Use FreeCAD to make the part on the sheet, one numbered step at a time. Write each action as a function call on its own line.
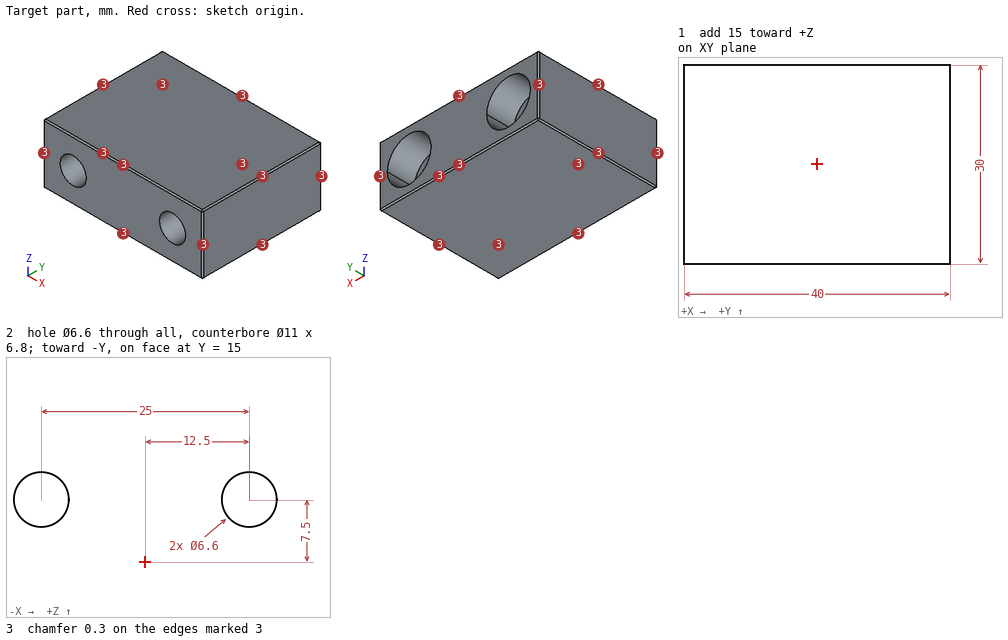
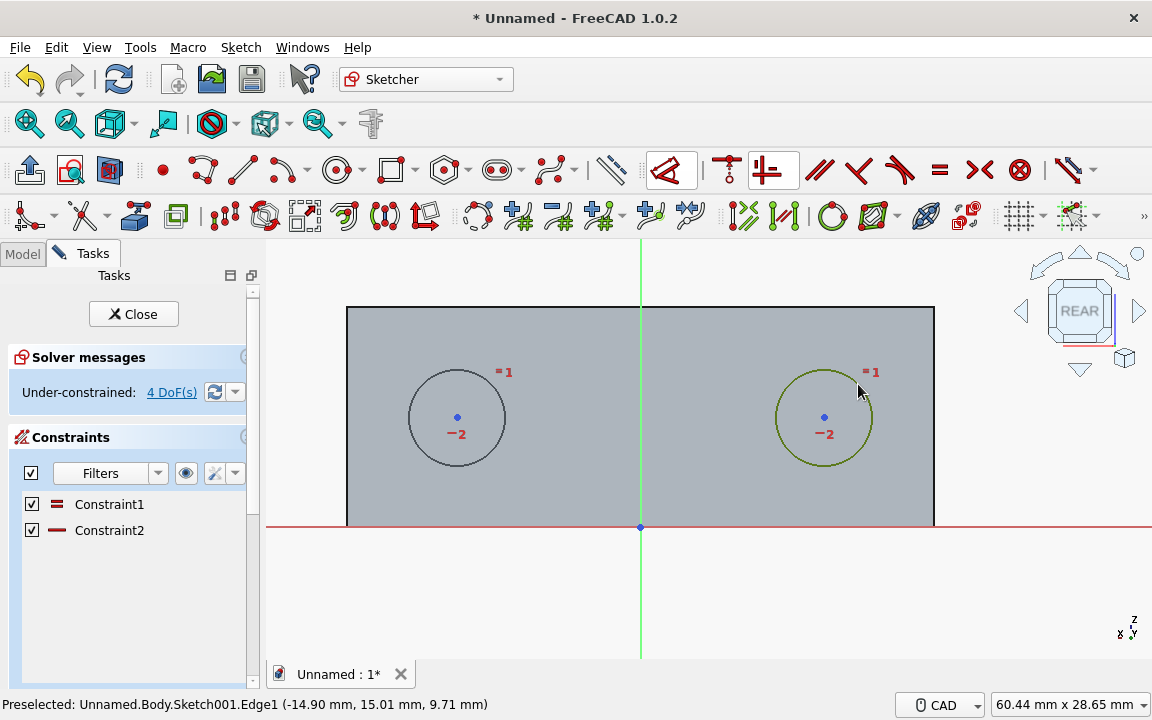
key(k)
key(o)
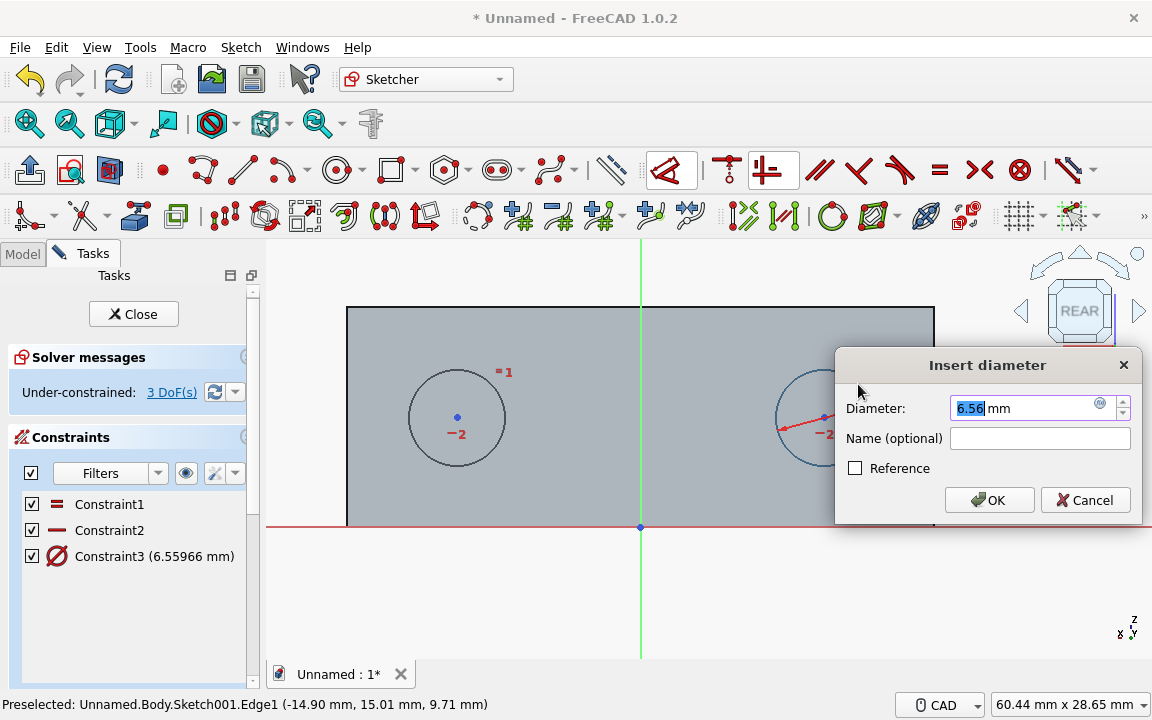
text(6.6)
key(Return)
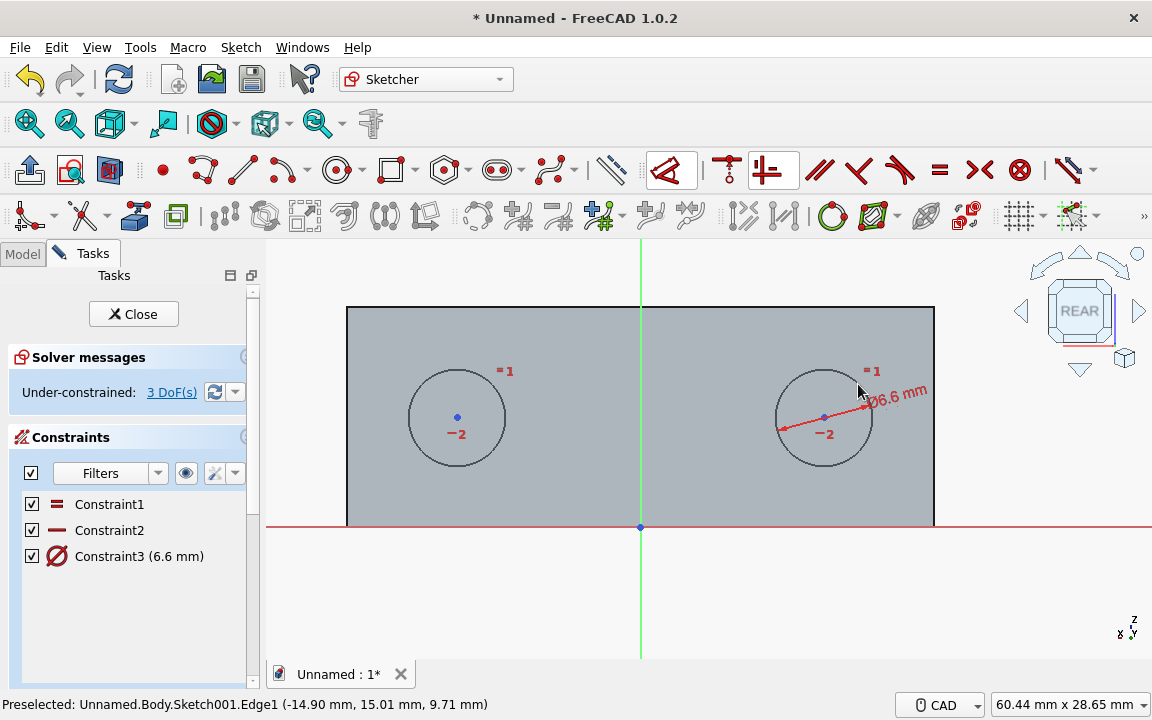
click(824, 418)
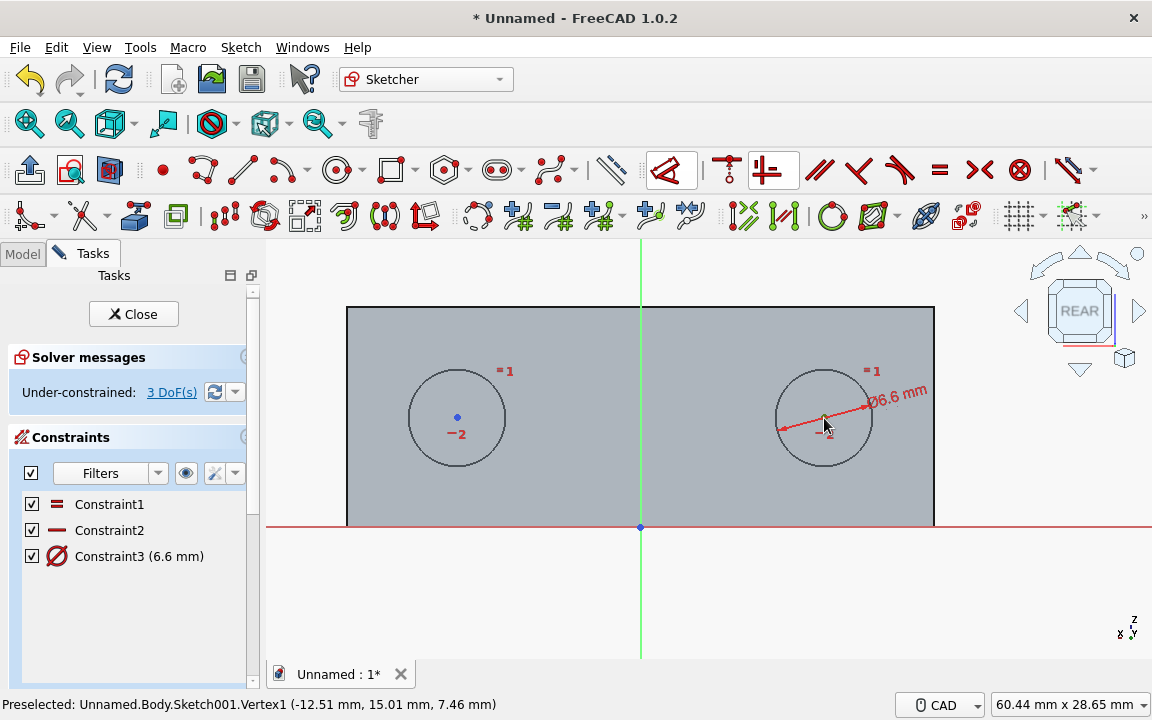
click(692, 170)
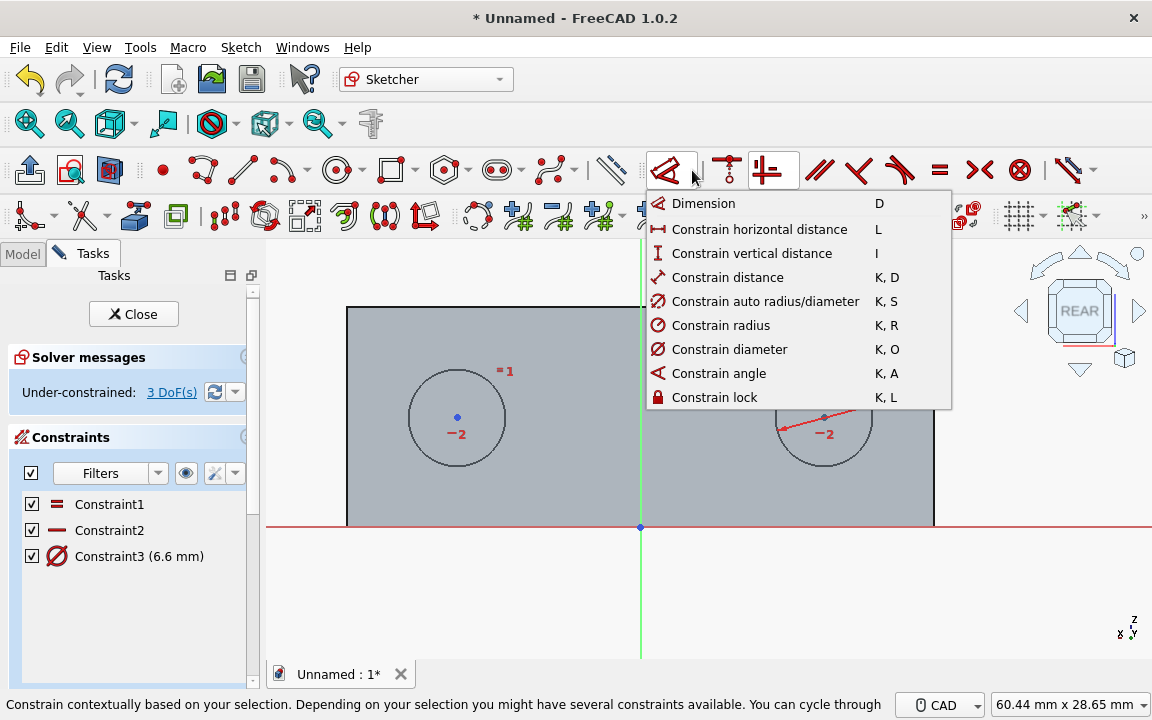
click(799, 253)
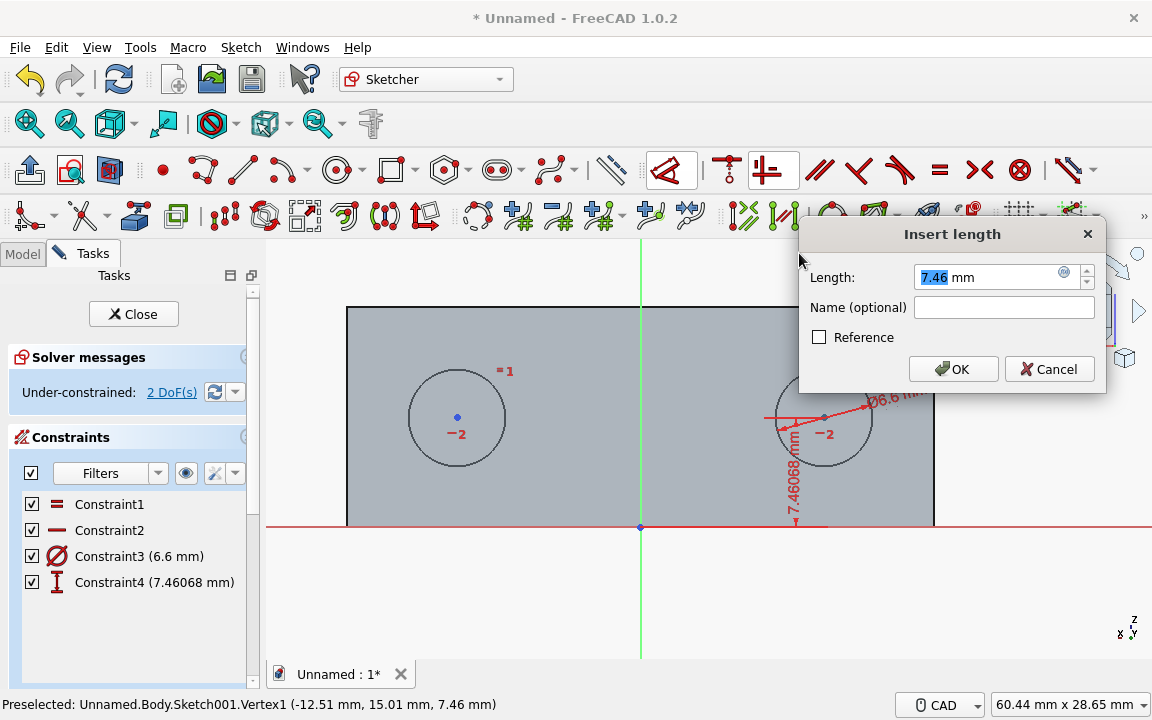
text(7.5)
key(Return)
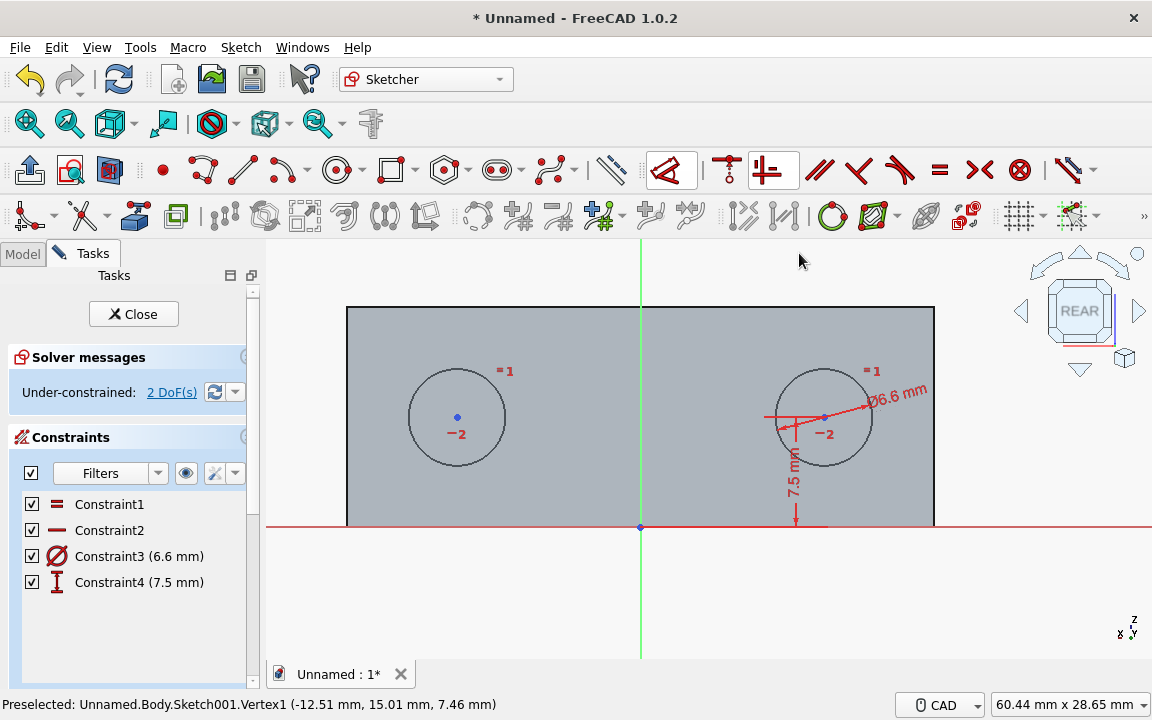
click(824, 417)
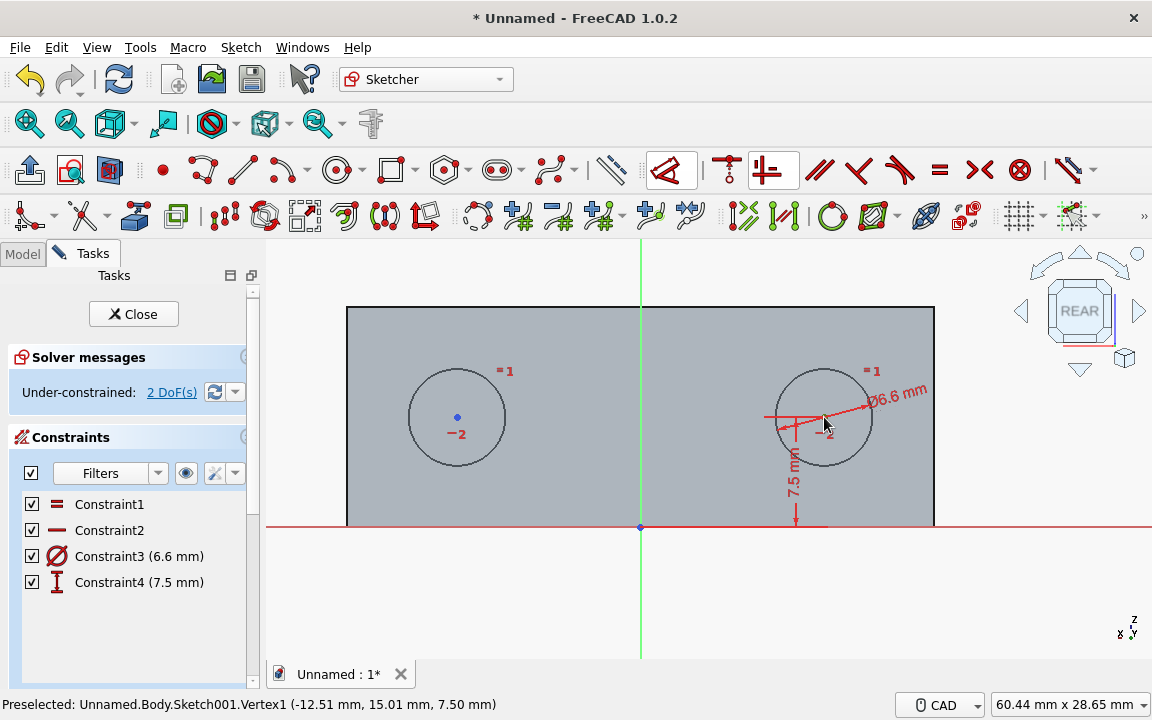
click(457, 417)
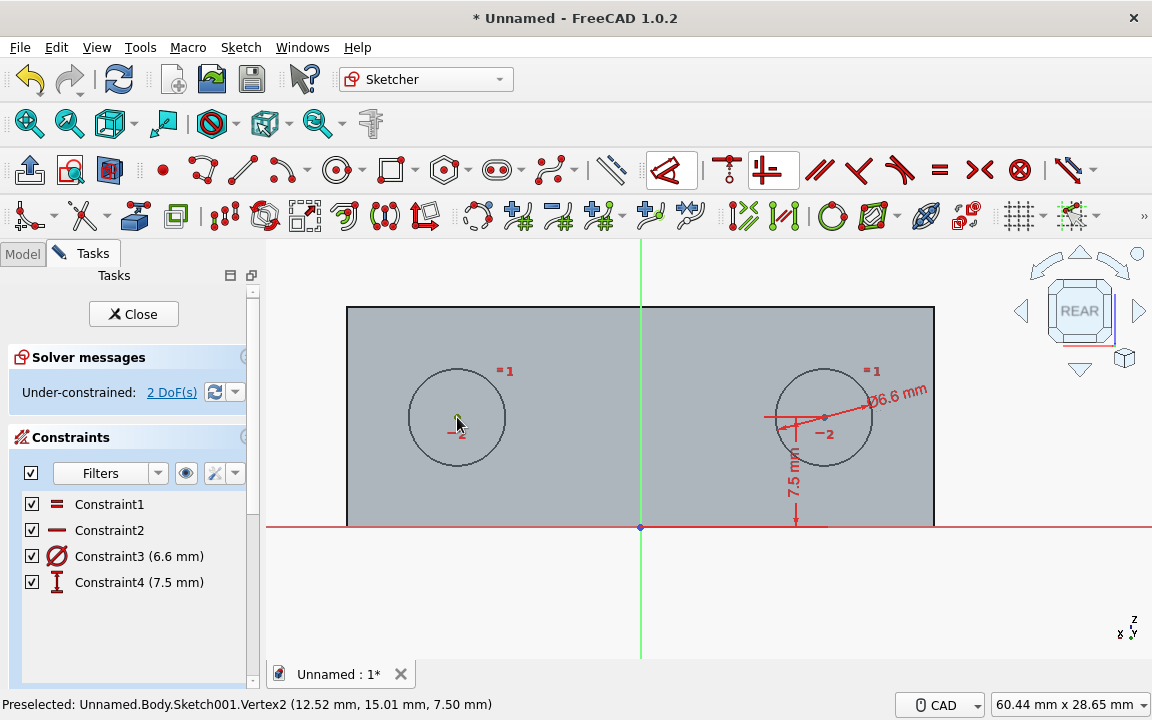
click(692, 170)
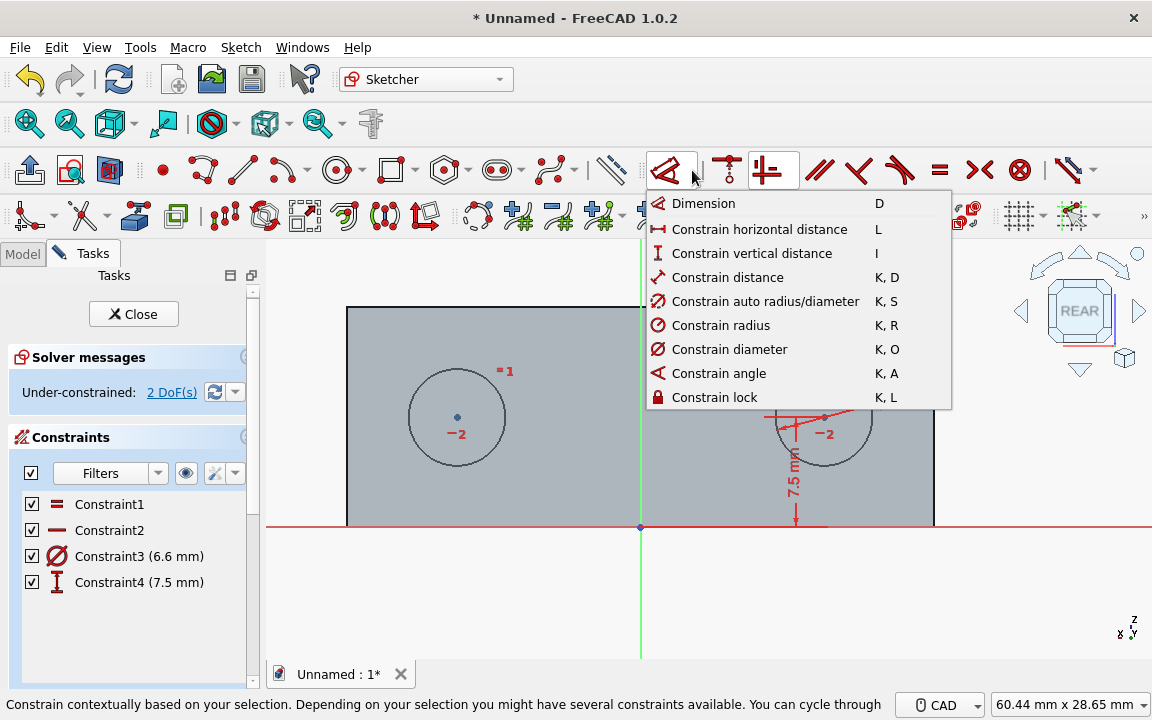
click(799, 229)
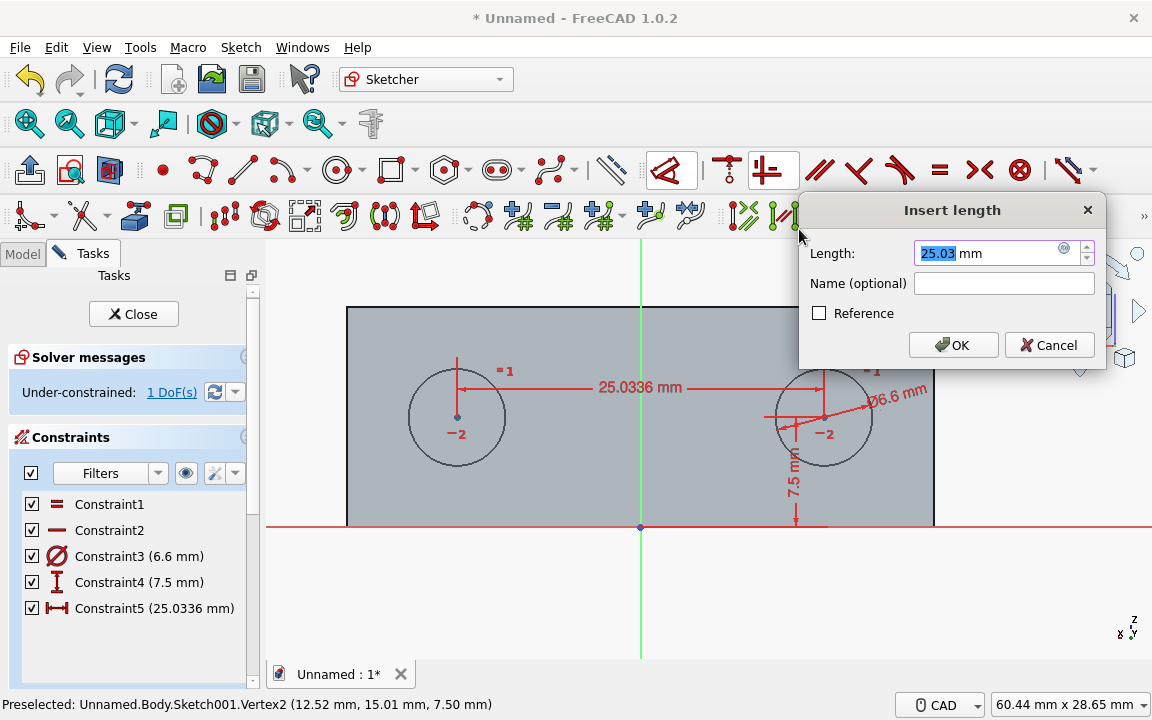
text(25)
key(Return)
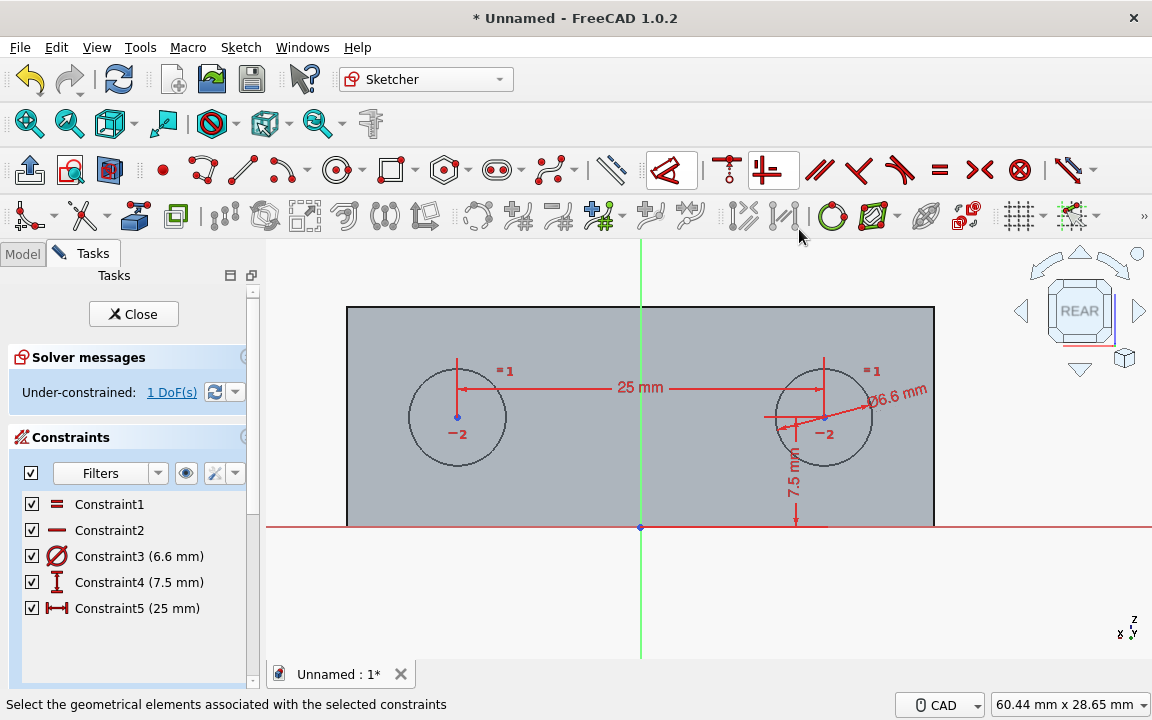
click(824, 417)